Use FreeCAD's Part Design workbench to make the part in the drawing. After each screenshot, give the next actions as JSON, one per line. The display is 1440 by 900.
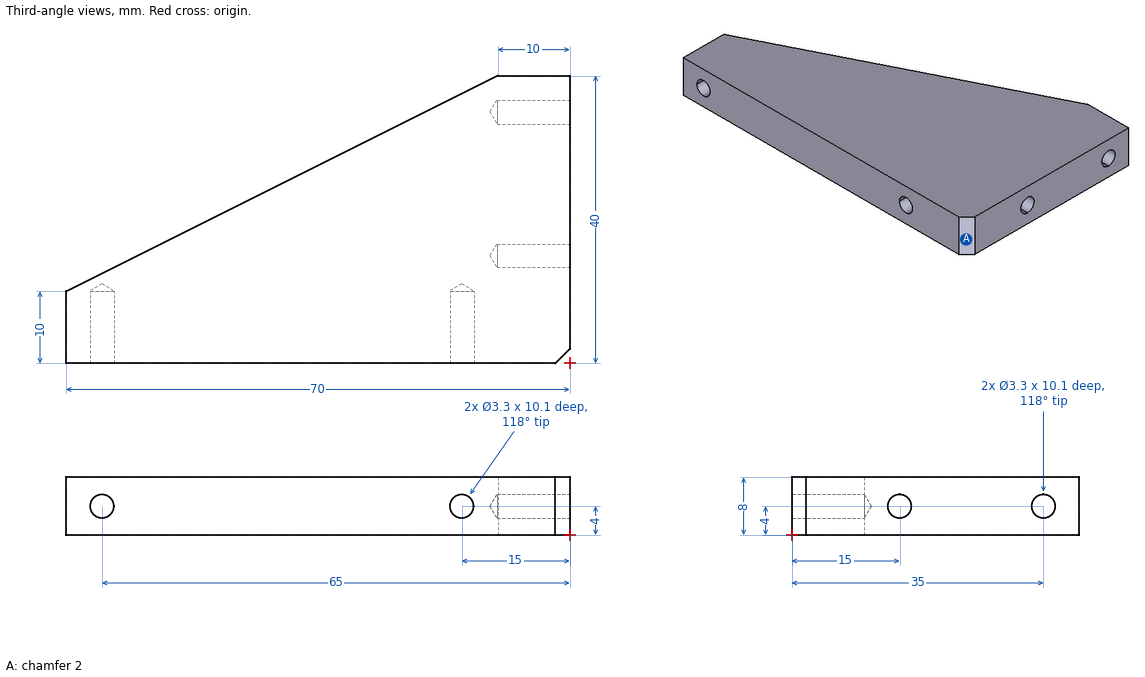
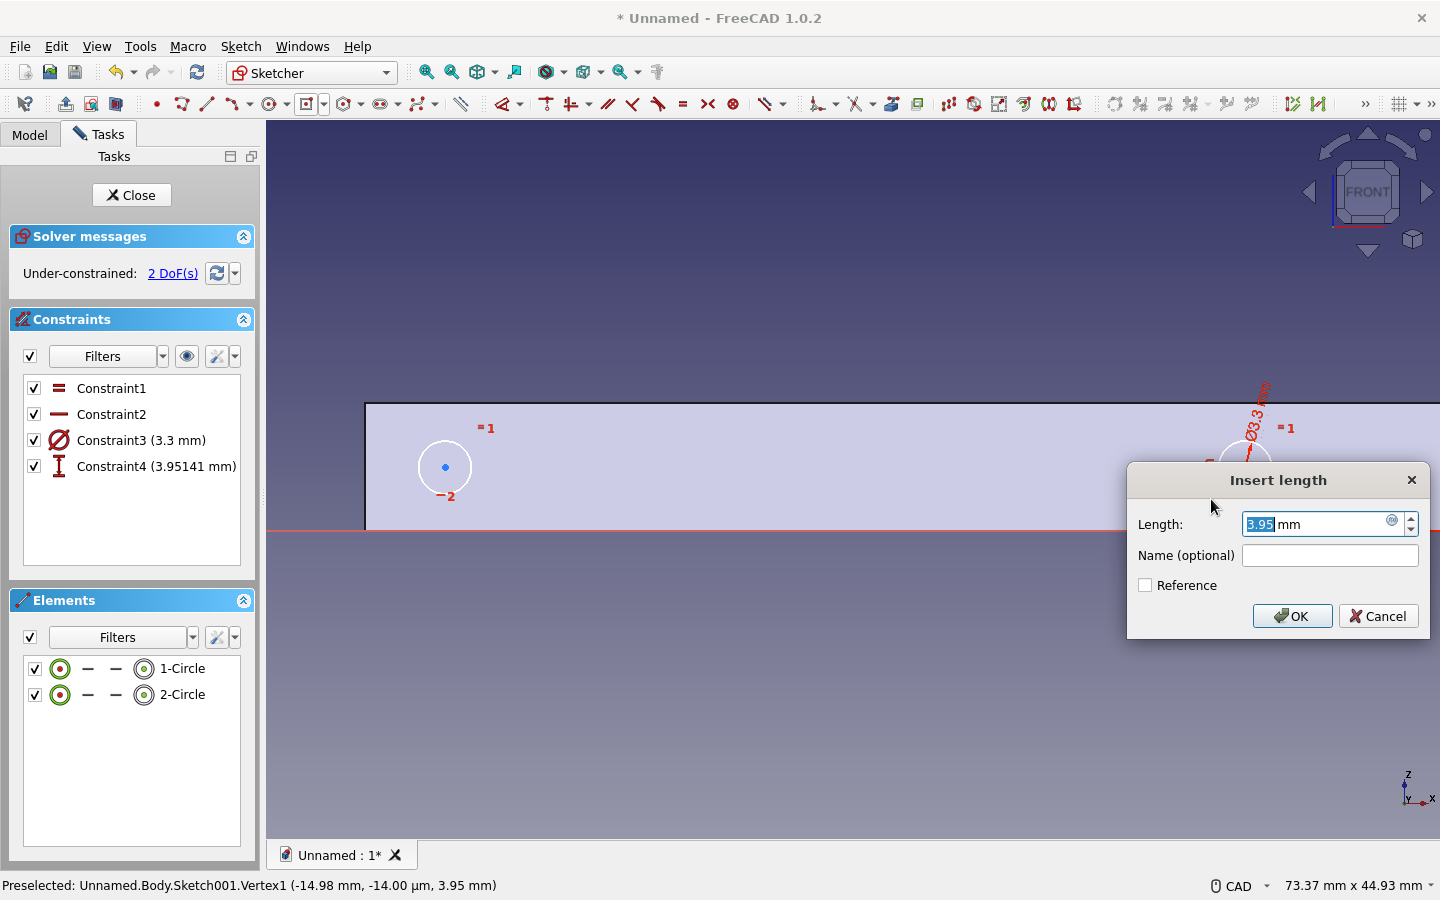
{"action": "type", "text": "4"}
{"action": "key", "text": "Return"}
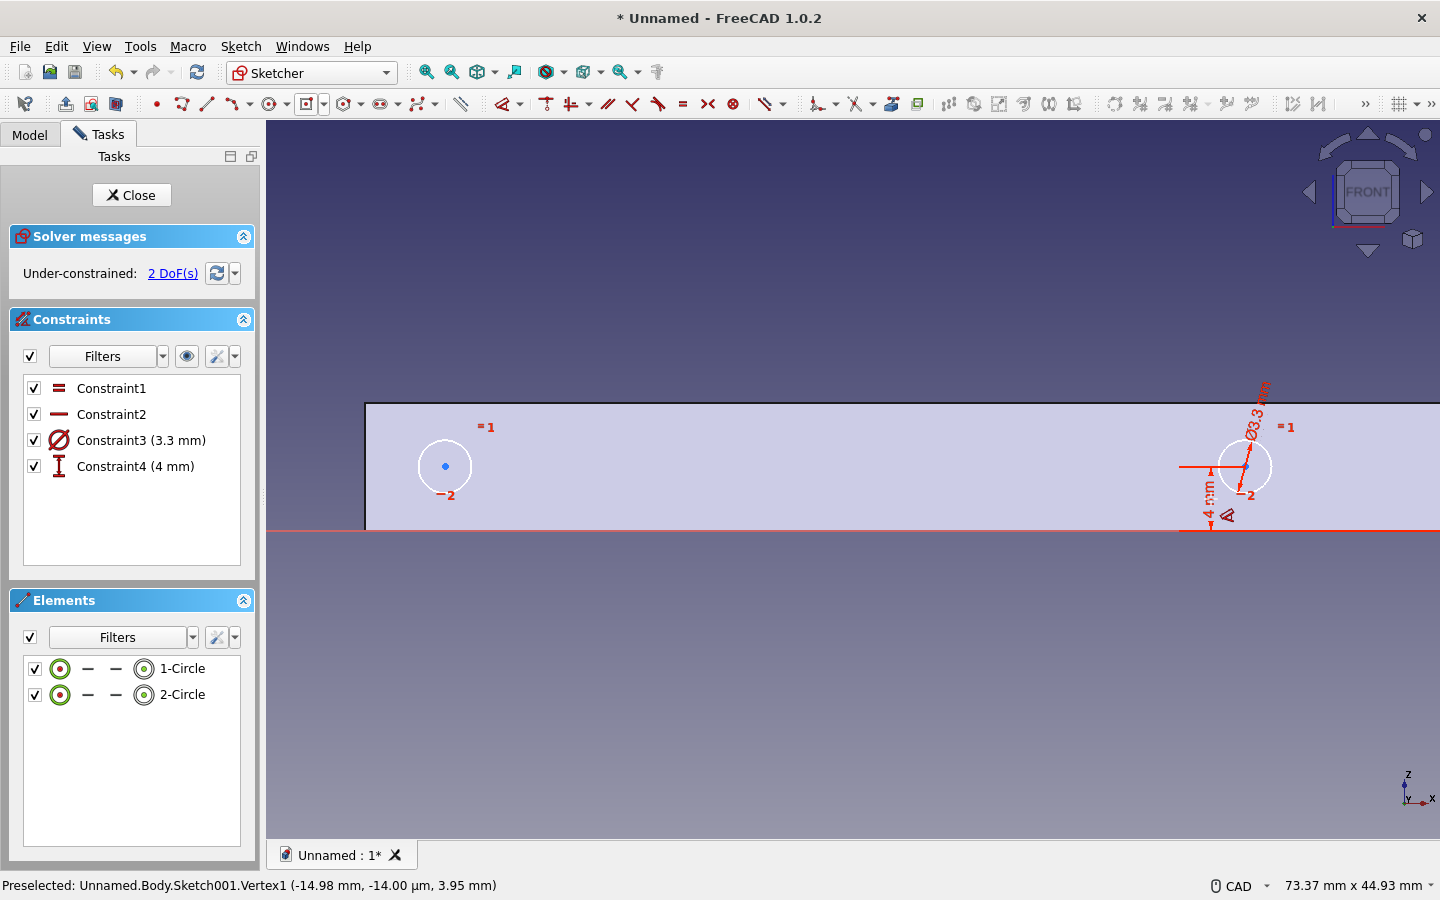
{"action": "left_click", "coordinate": [1245, 467]}
{"action": "left_click", "coordinate": [1260, 565]}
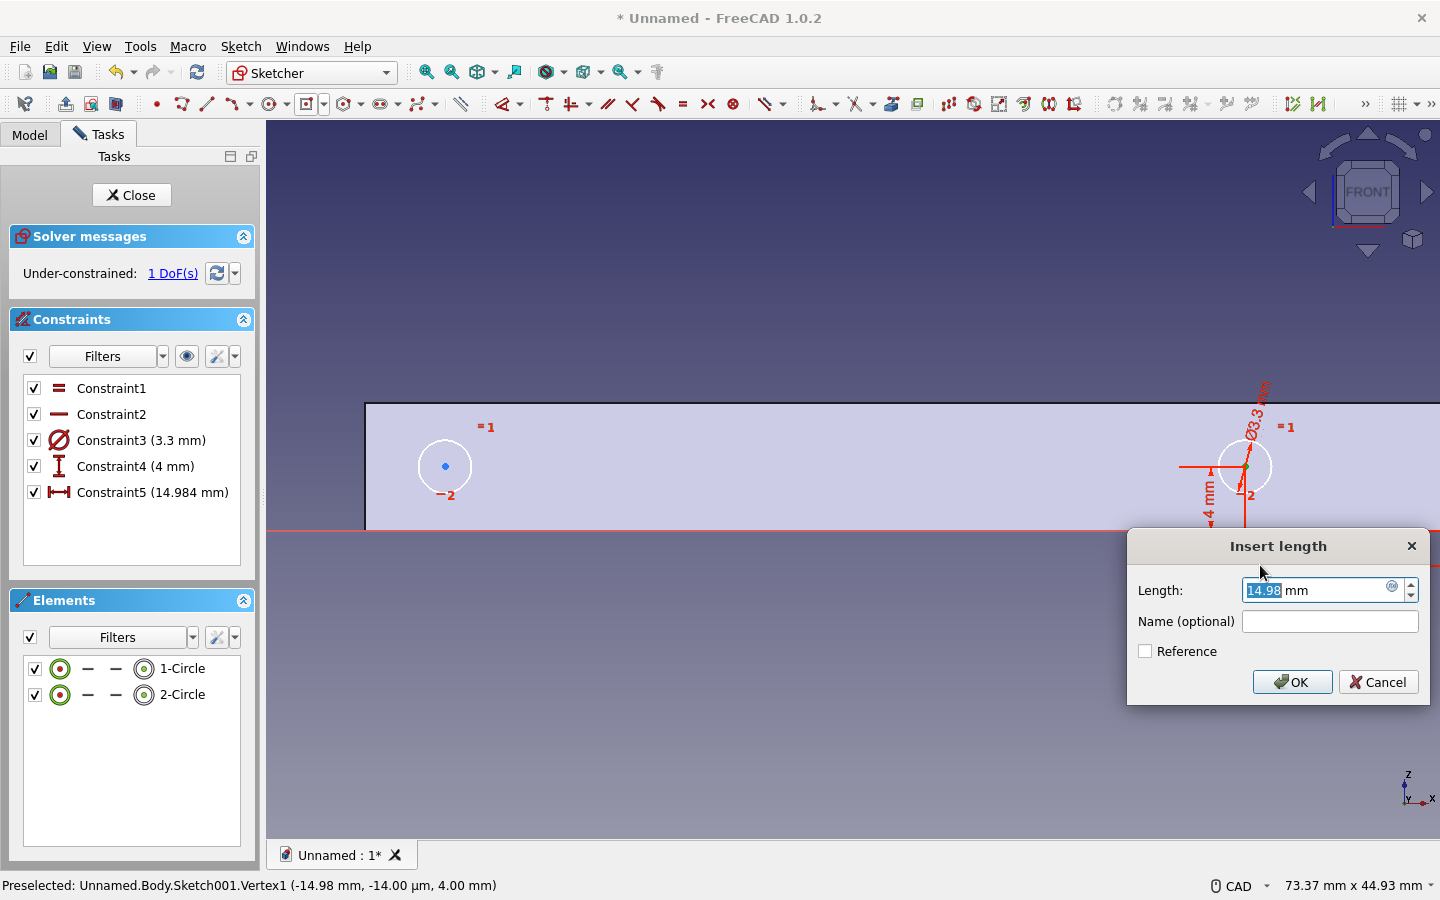
{"action": "type", "text": "15"}
{"action": "key", "text": "Return"}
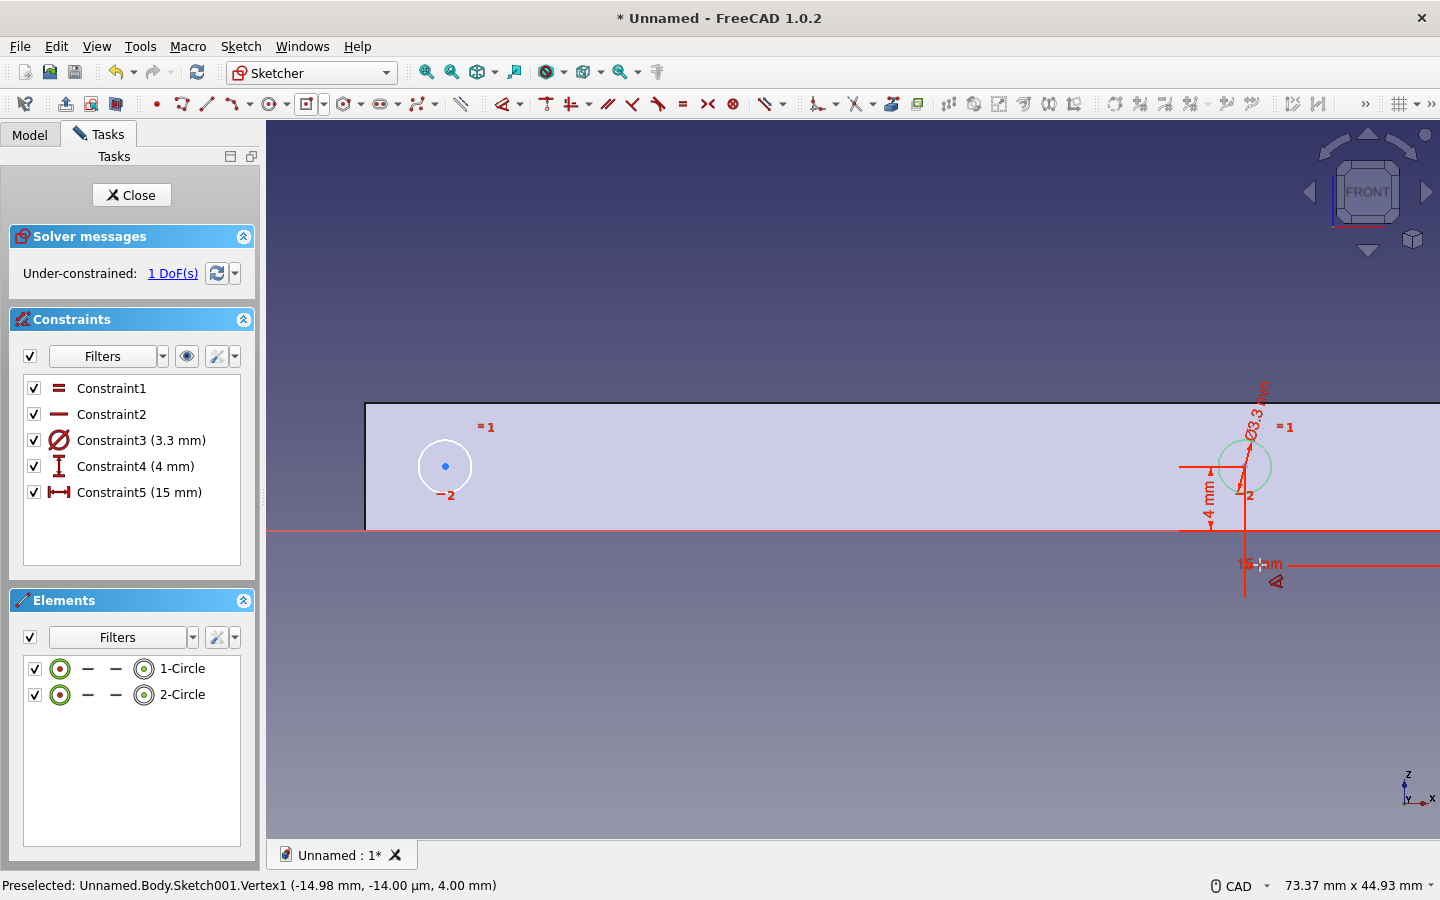
{"action": "left_click", "coordinate": [445, 467]}
{"action": "left_click", "coordinate": [860, 565]}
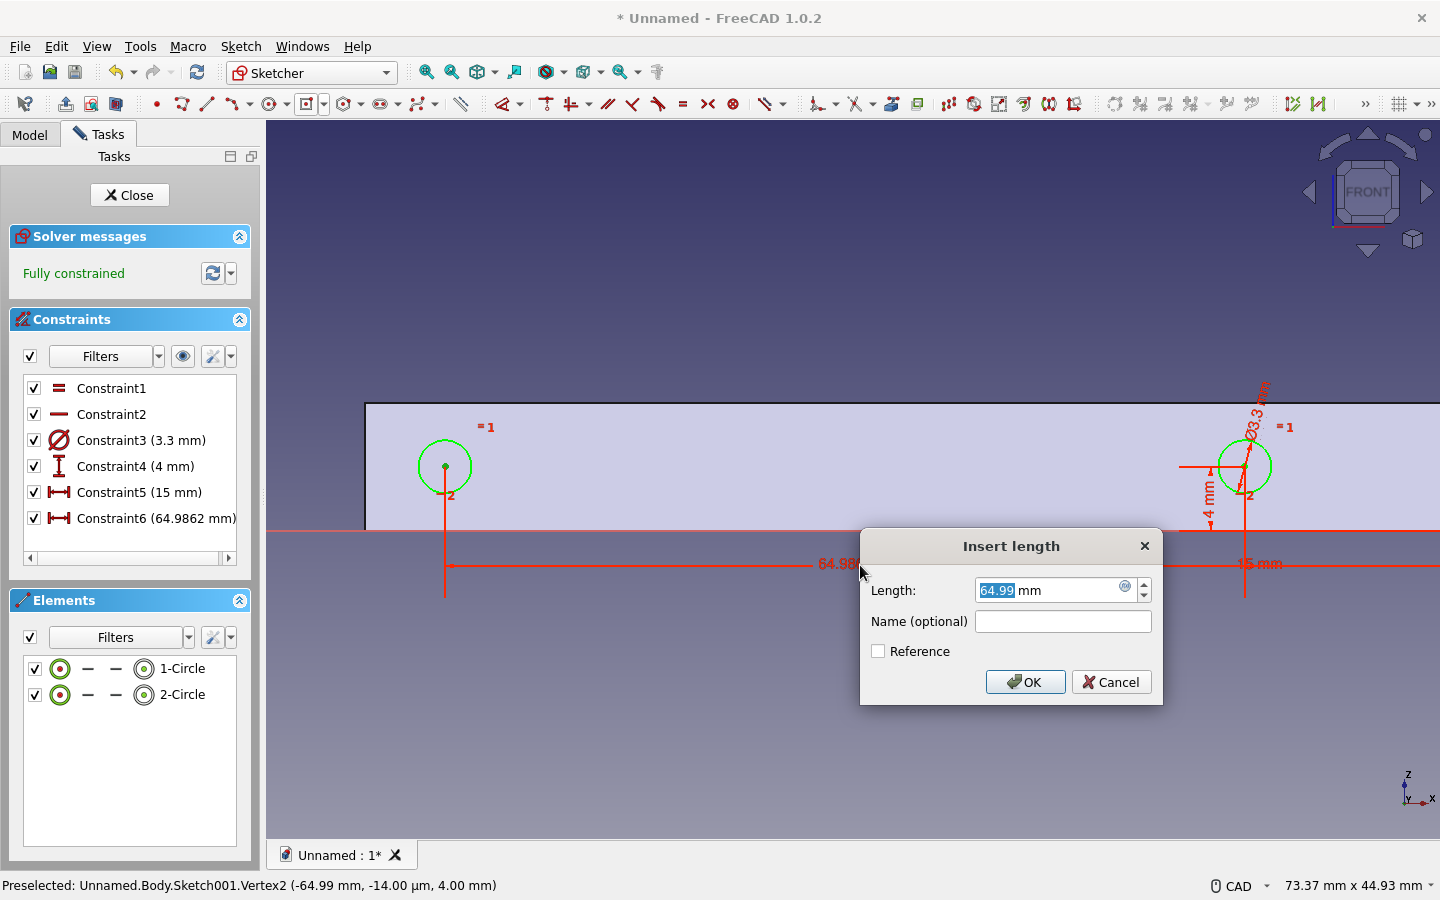
{"action": "type", "text": "65"}
{"action": "key", "text": "Return"}
{"action": "key", "text": "Escape"}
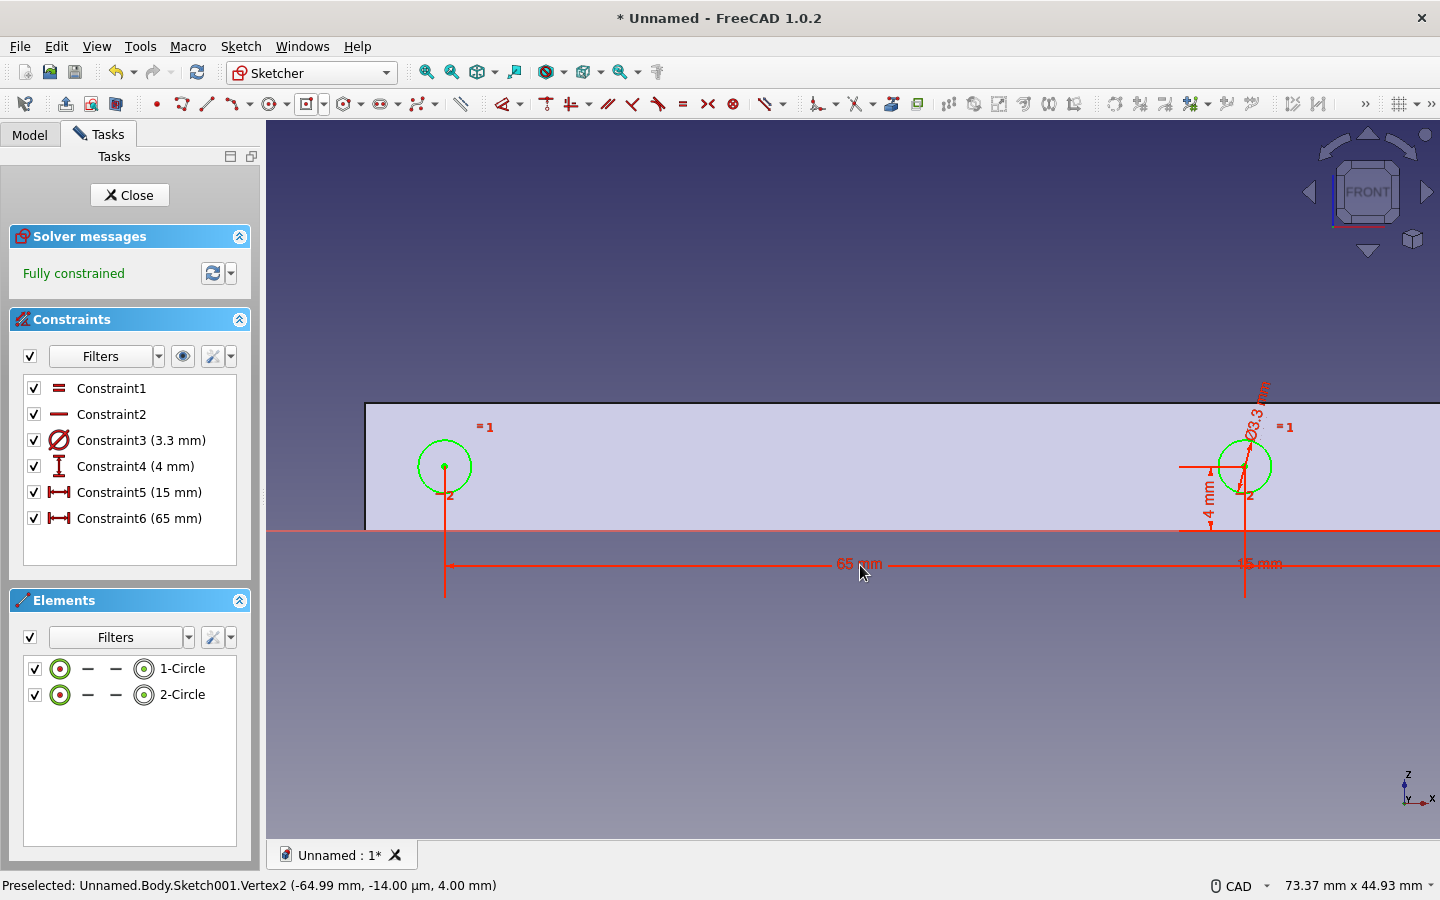
{"action": "left_click", "coordinate": [130, 195]}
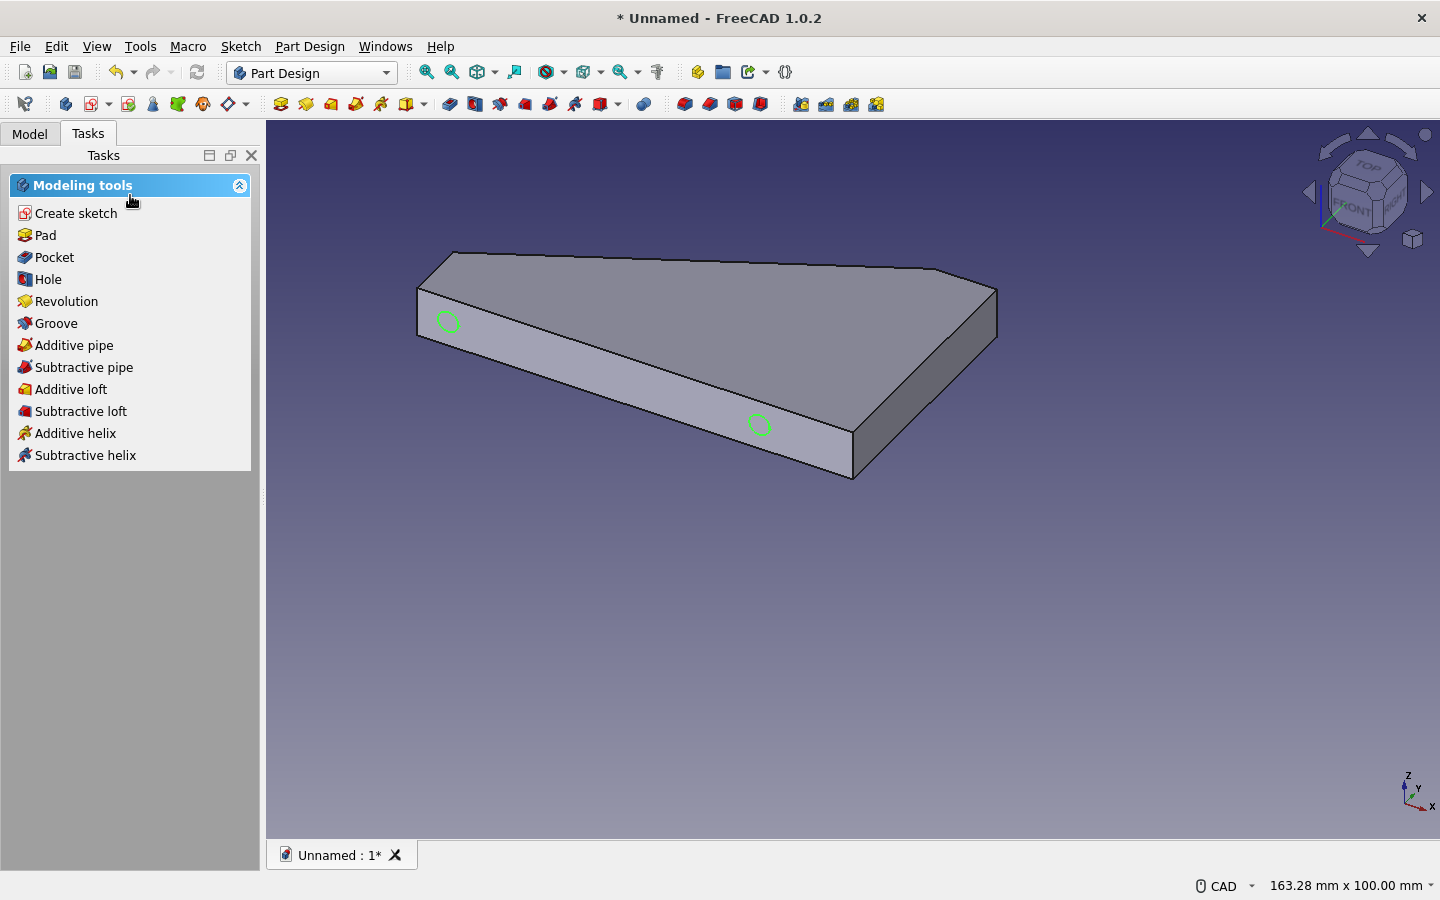
{"action": "left_click", "coordinate": [475, 104]}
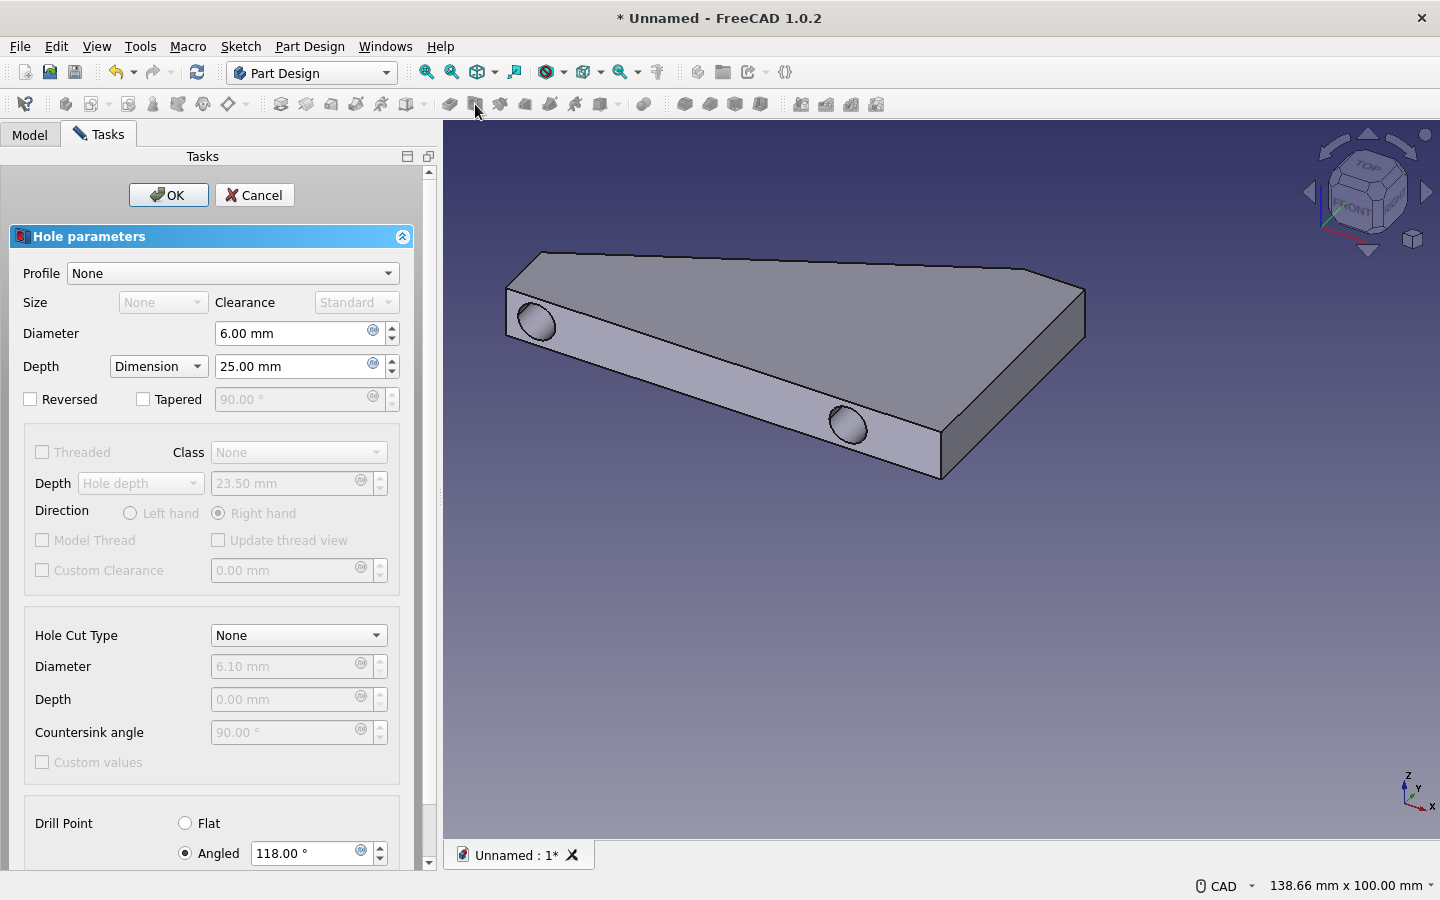
{"action": "triple_click", "coordinate": [300, 334]}